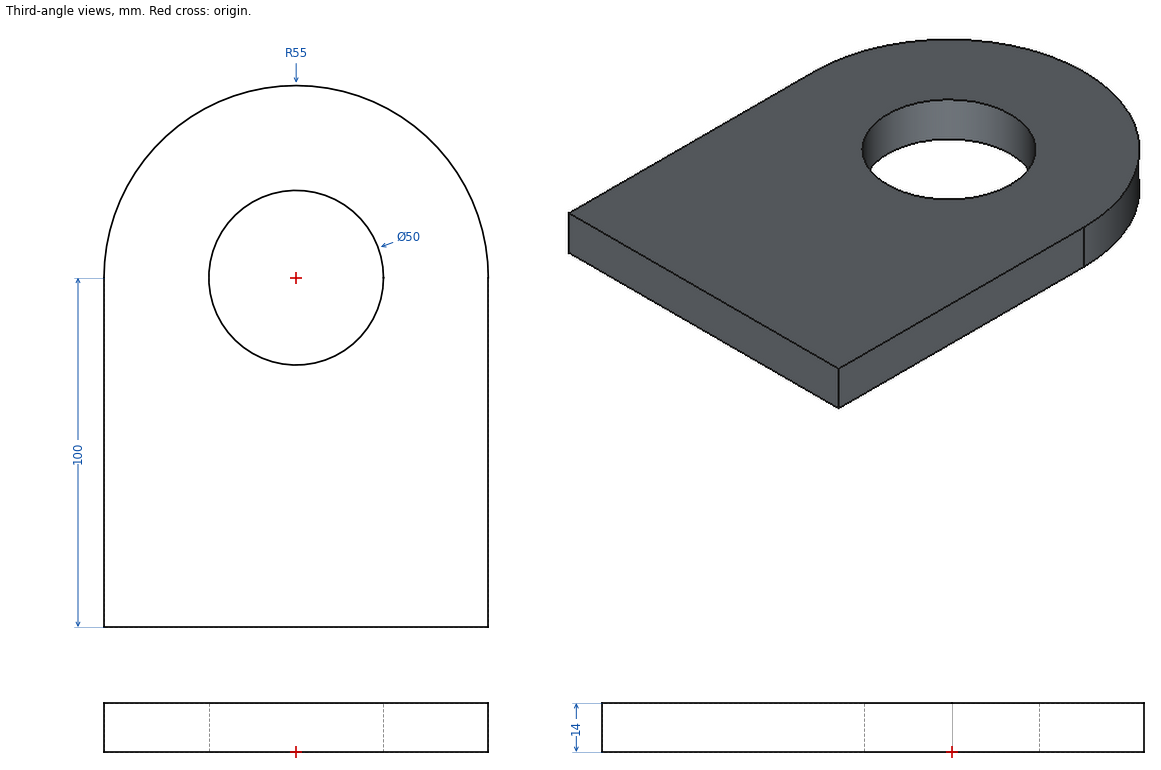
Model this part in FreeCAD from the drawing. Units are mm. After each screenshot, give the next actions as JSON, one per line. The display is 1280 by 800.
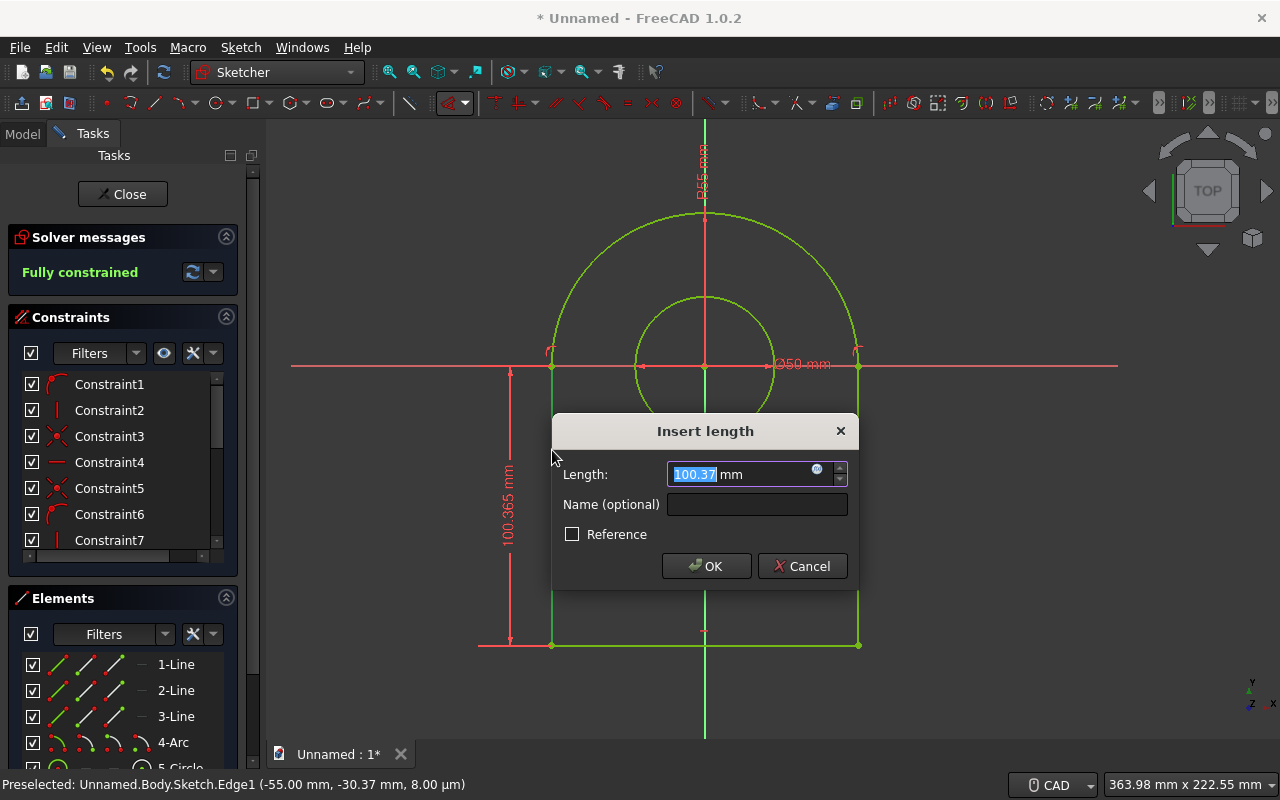
{"action": "type", "text": "100"}
{"action": "key", "text": "Return"}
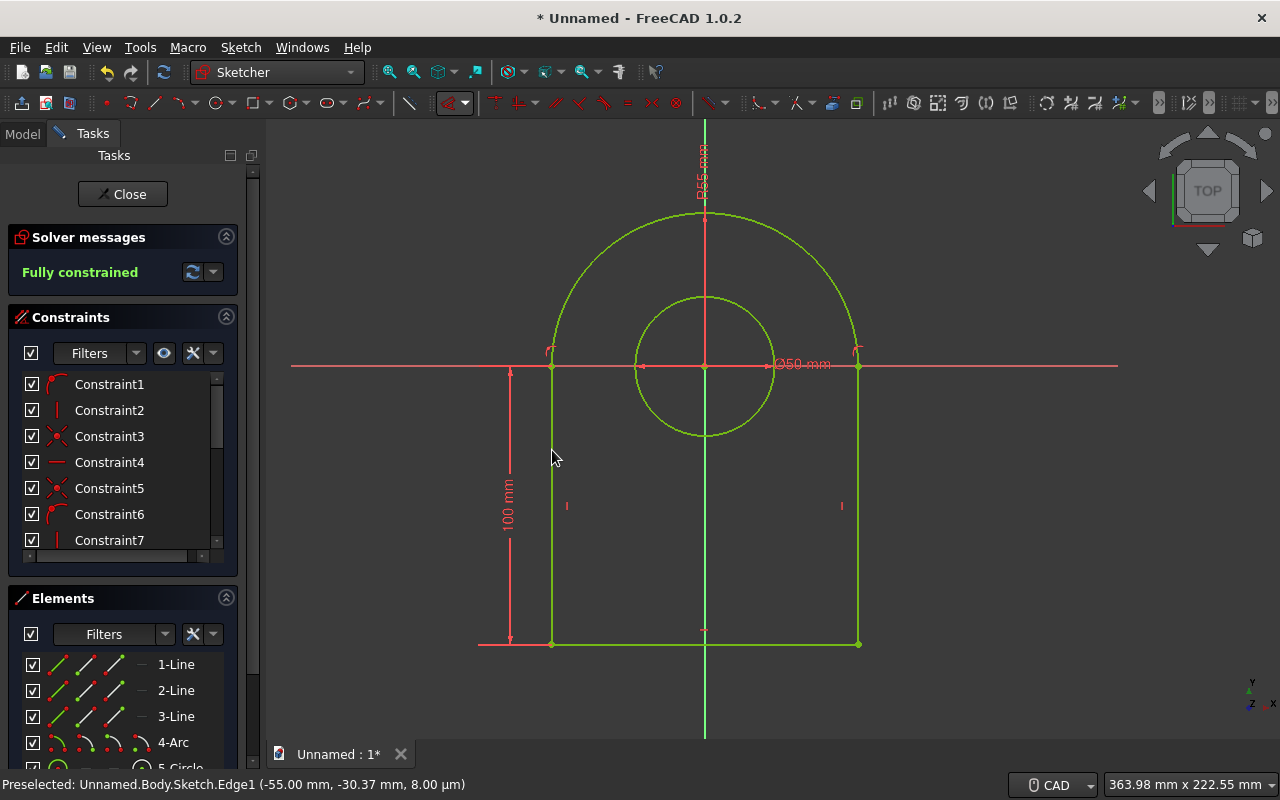
{"action": "left_click", "coordinate": [123, 194]}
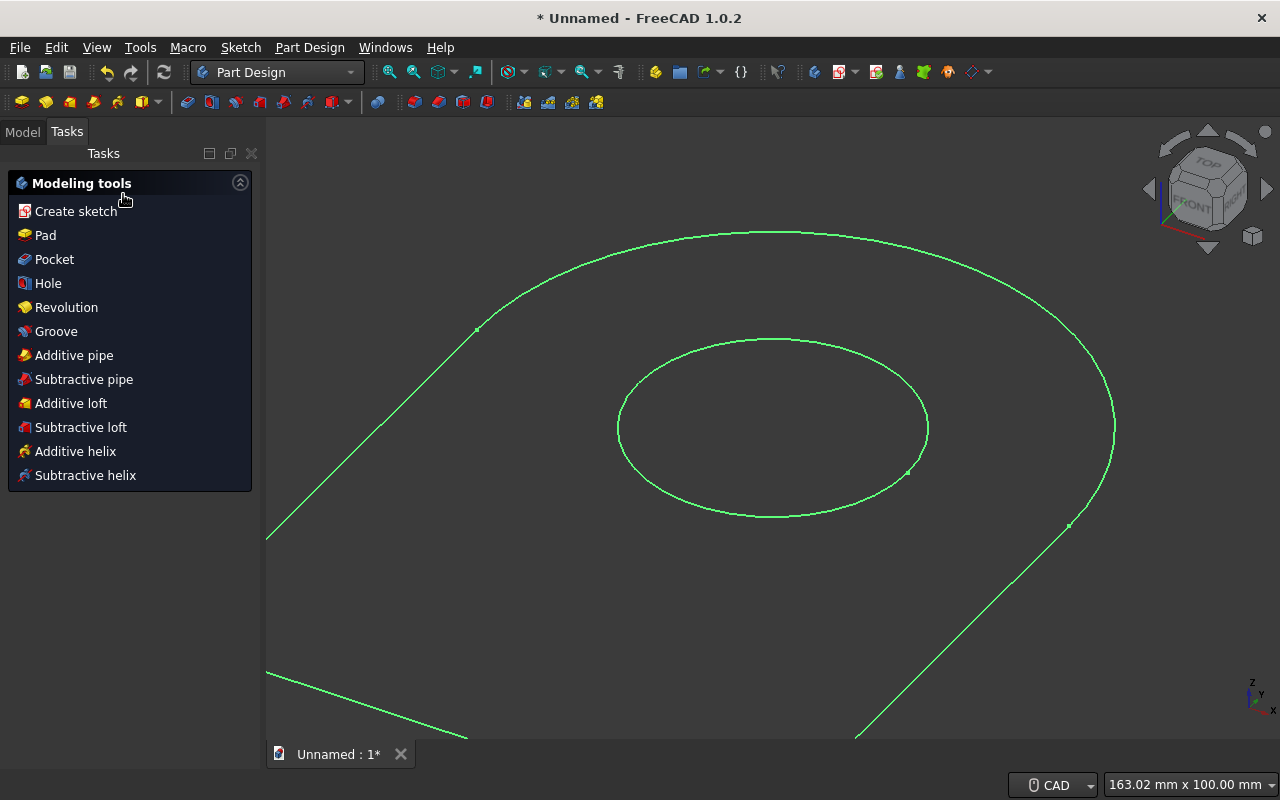
{"action": "left_click", "coordinate": [22, 102]}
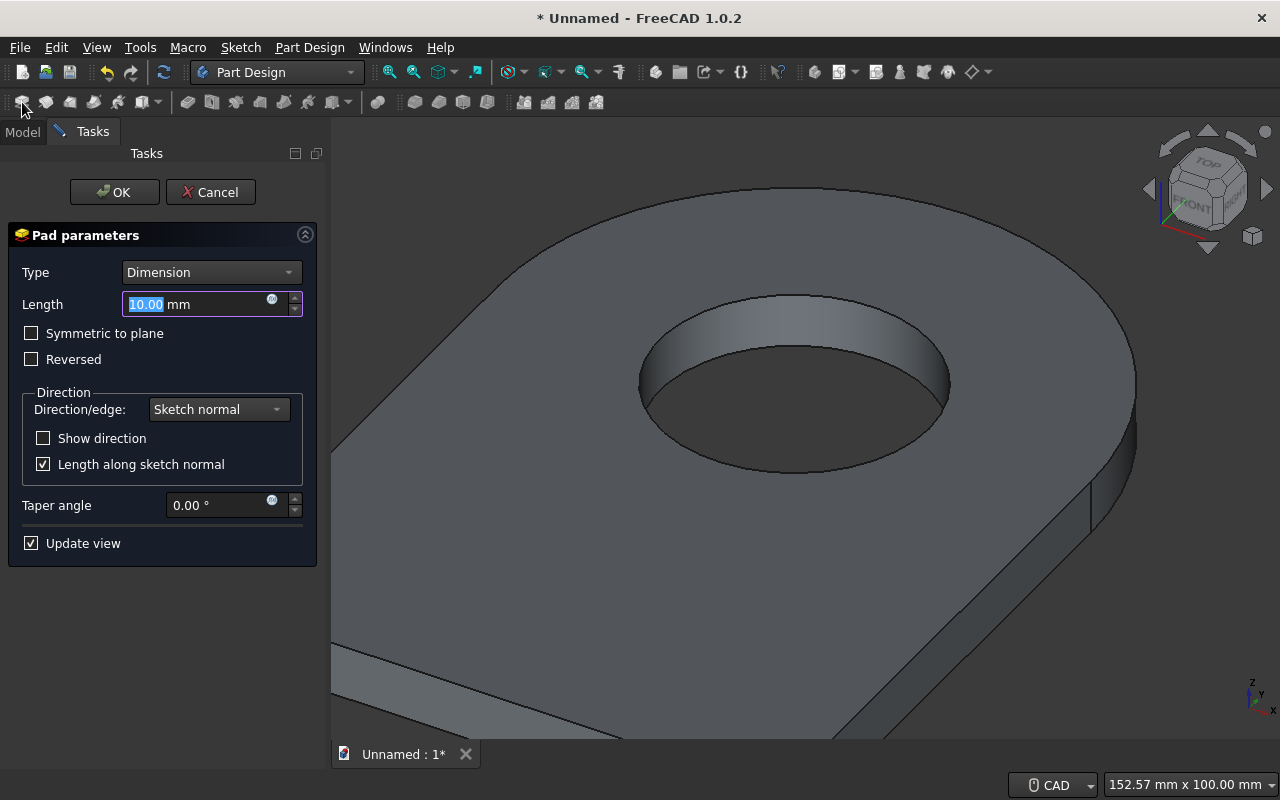
{"action": "type", "text": "14"}
{"action": "key", "text": "Tab"}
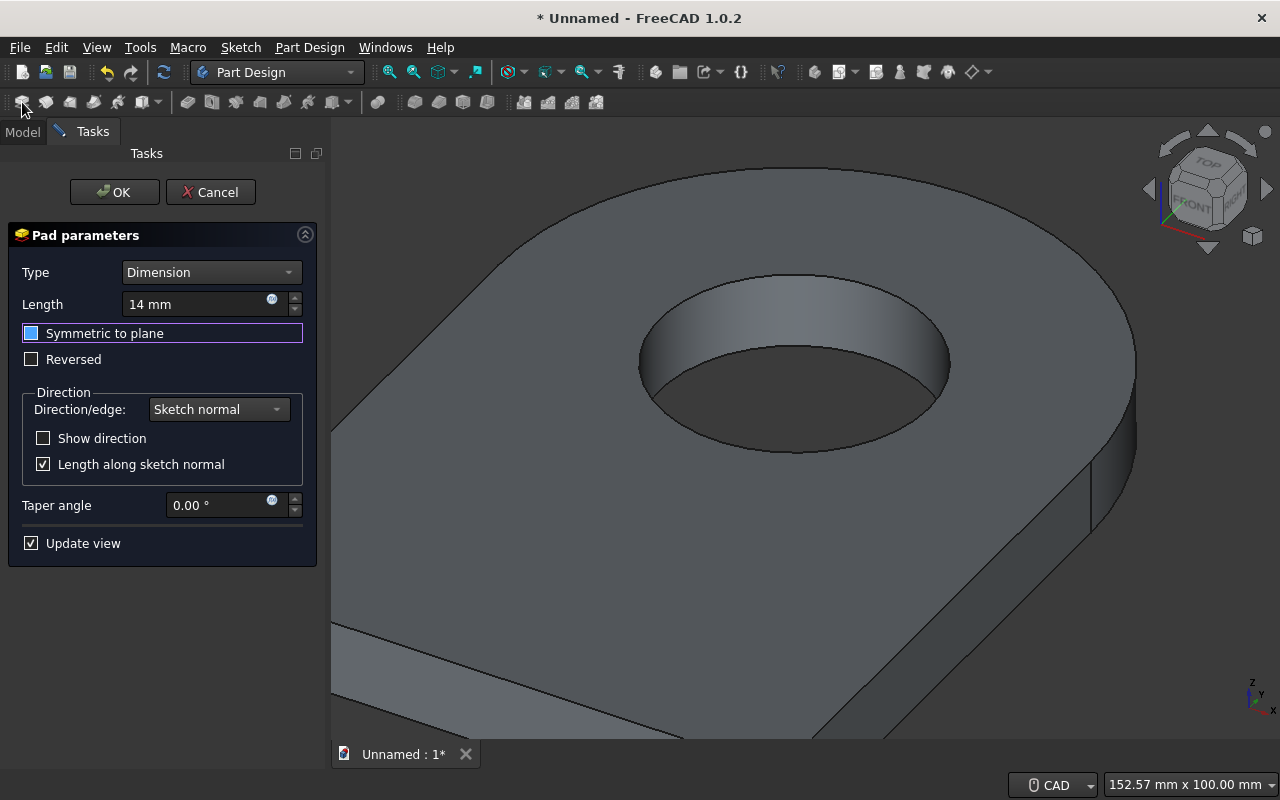
{"action": "left_click", "coordinate": [115, 192]}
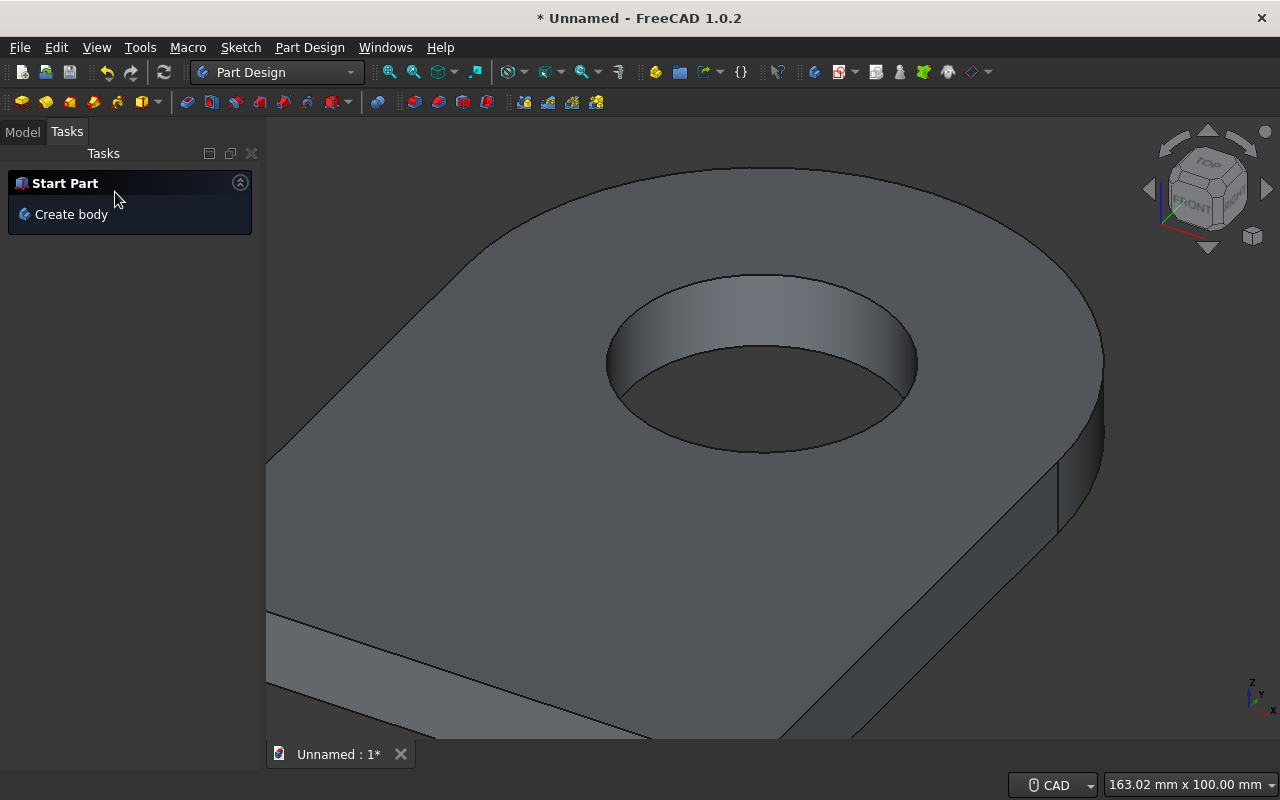
{"action": "key", "text": "0"}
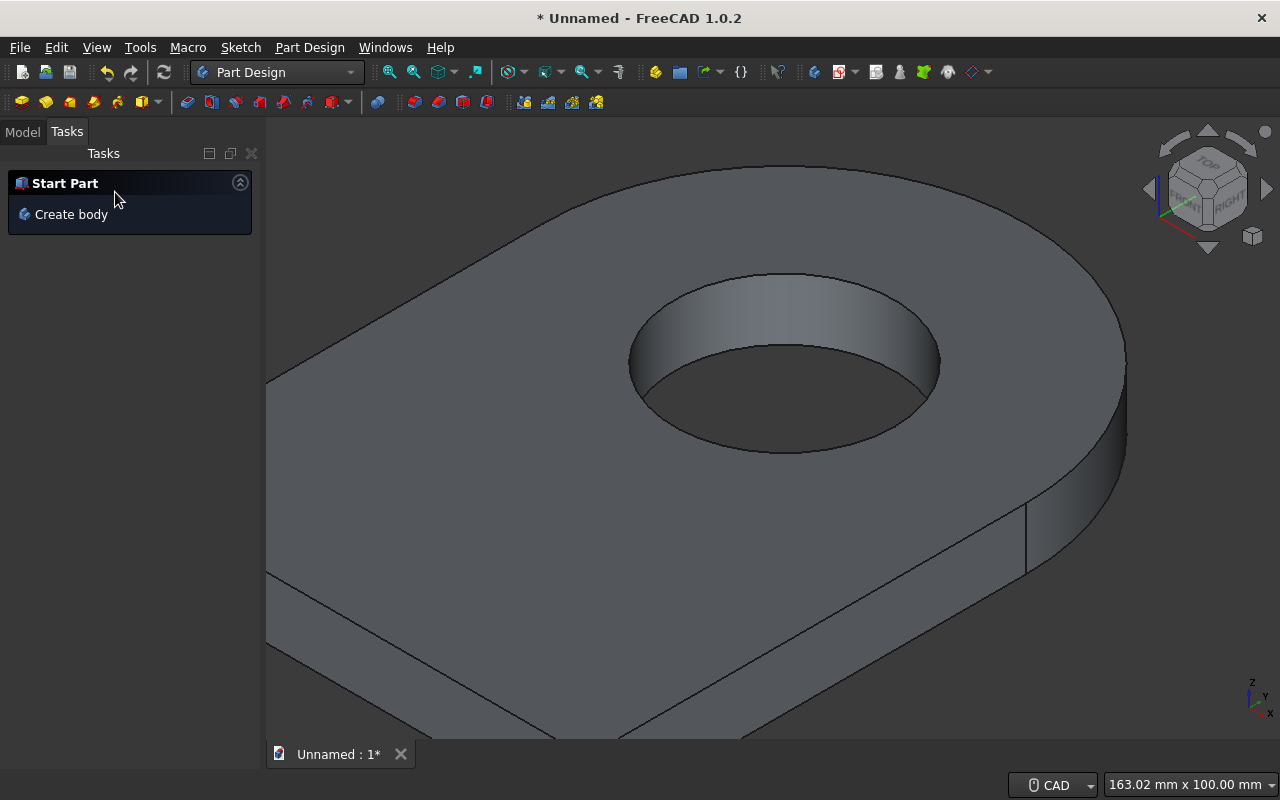
{"action": "left_click", "coordinate": [390, 72]}